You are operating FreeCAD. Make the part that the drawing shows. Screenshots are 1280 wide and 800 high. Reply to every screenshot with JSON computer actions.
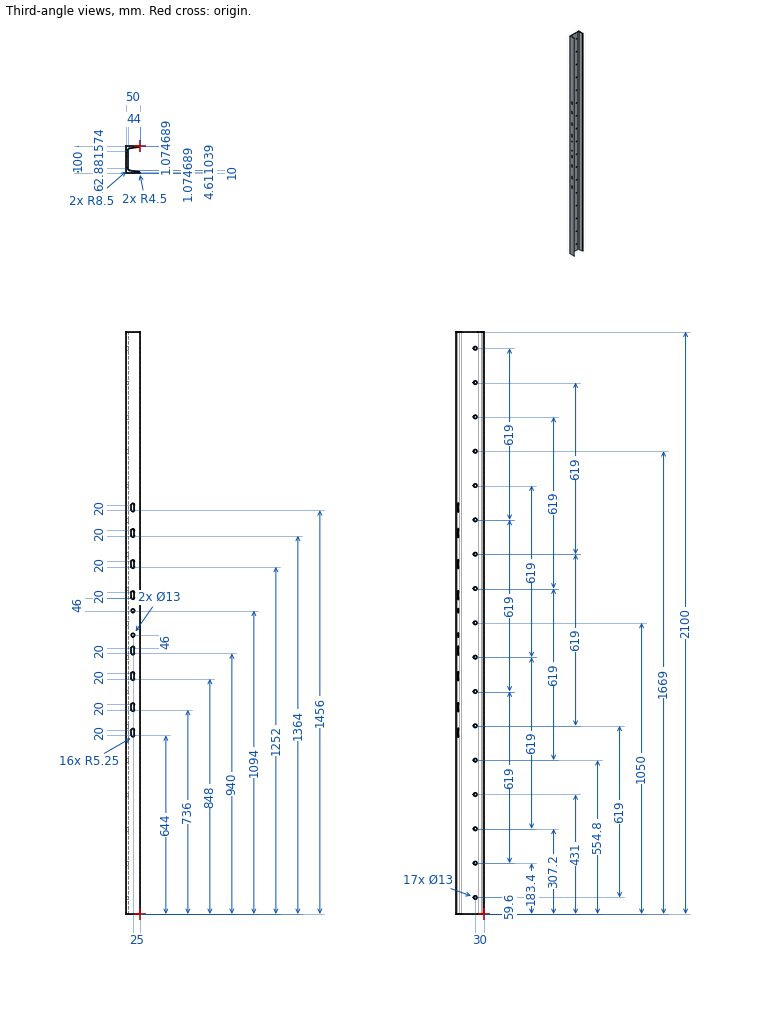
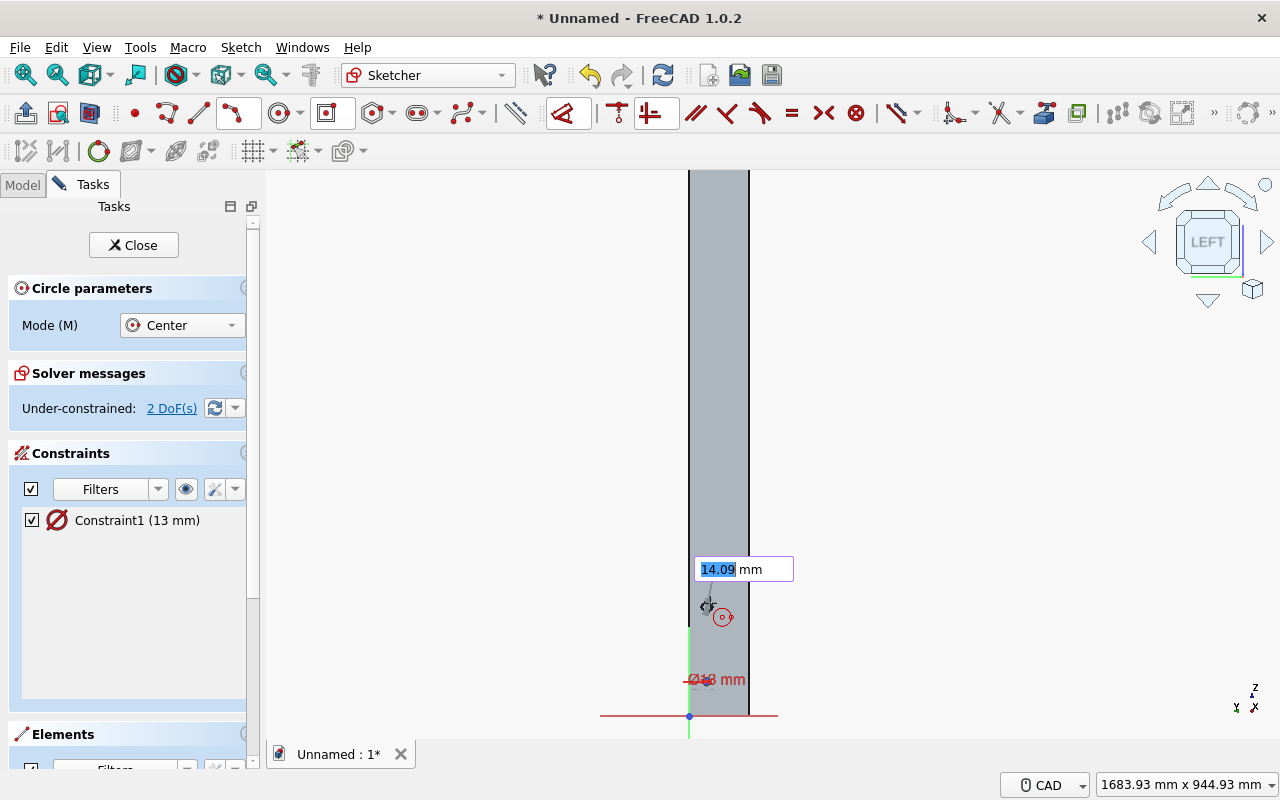
{"action": "type", "text": "13"}
{"action": "key", "text": "Return"}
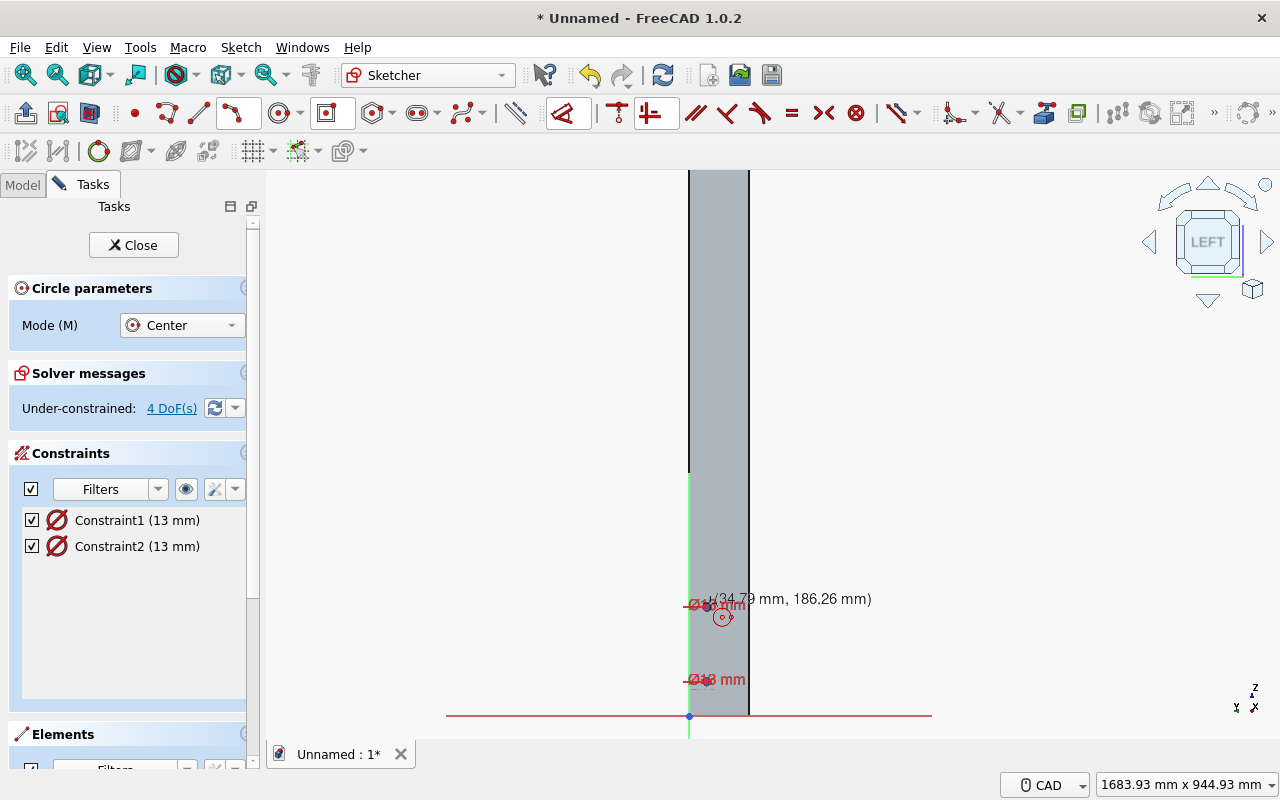
{"action": "scroll", "coordinate": [707, 531], "scroll_direction": "up", "scroll_amount": 9}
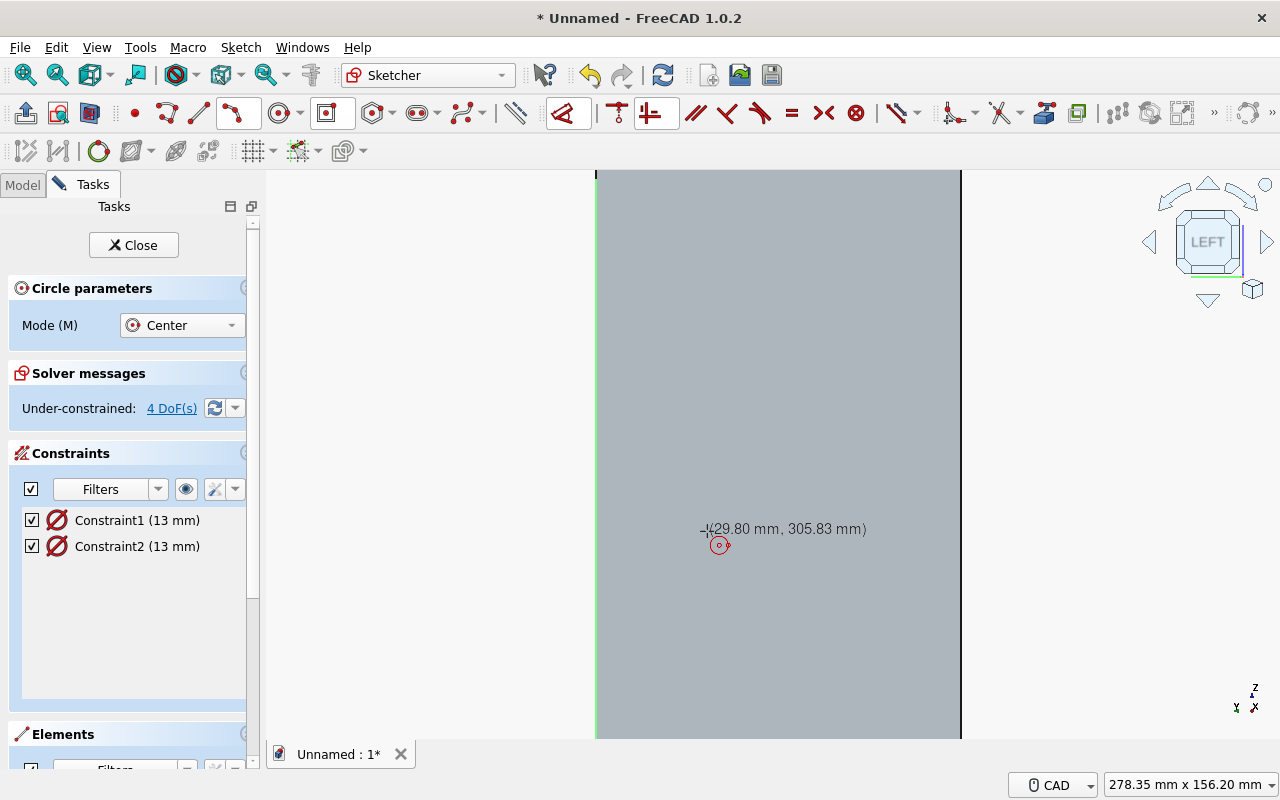
{"action": "scroll", "coordinate": [707, 587], "scroll_direction": "down", "scroll_amount": 15}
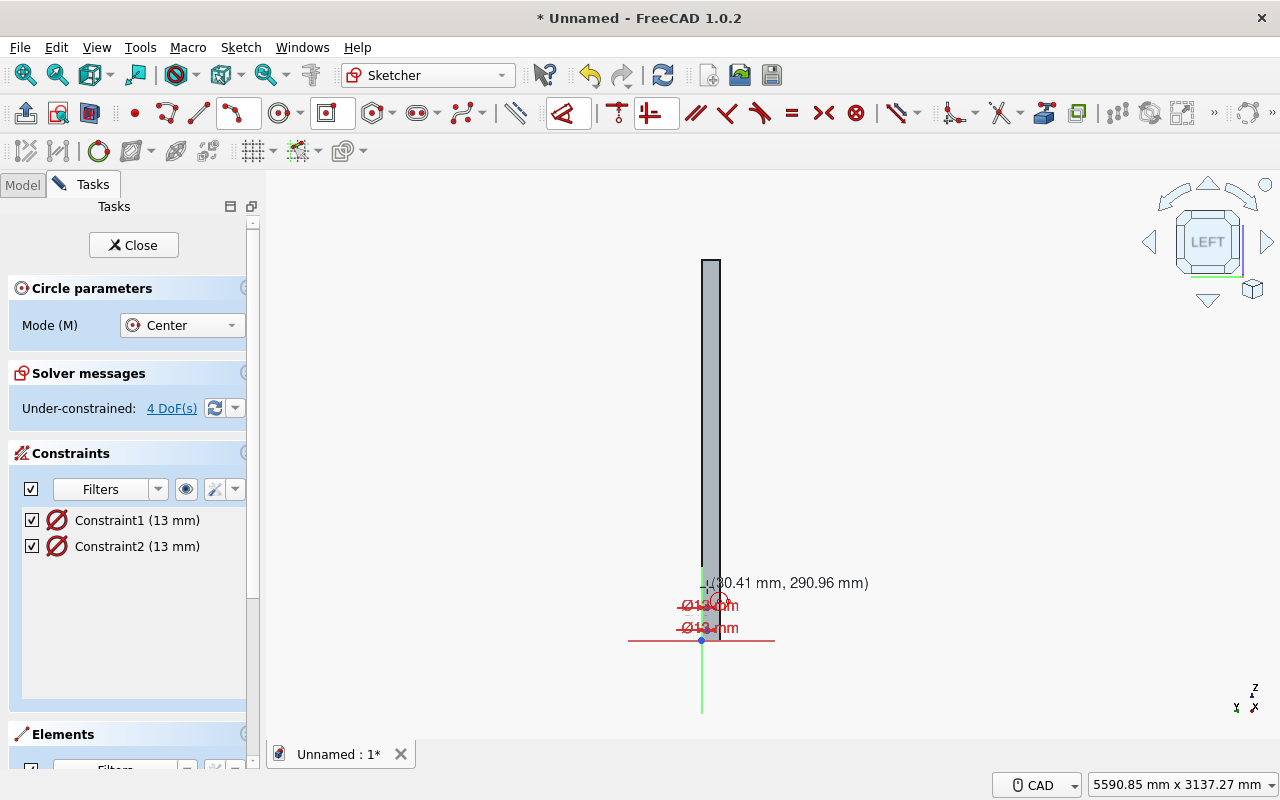
{"action": "scroll", "coordinate": [707, 585], "scroll_direction": "up", "scroll_amount": 6}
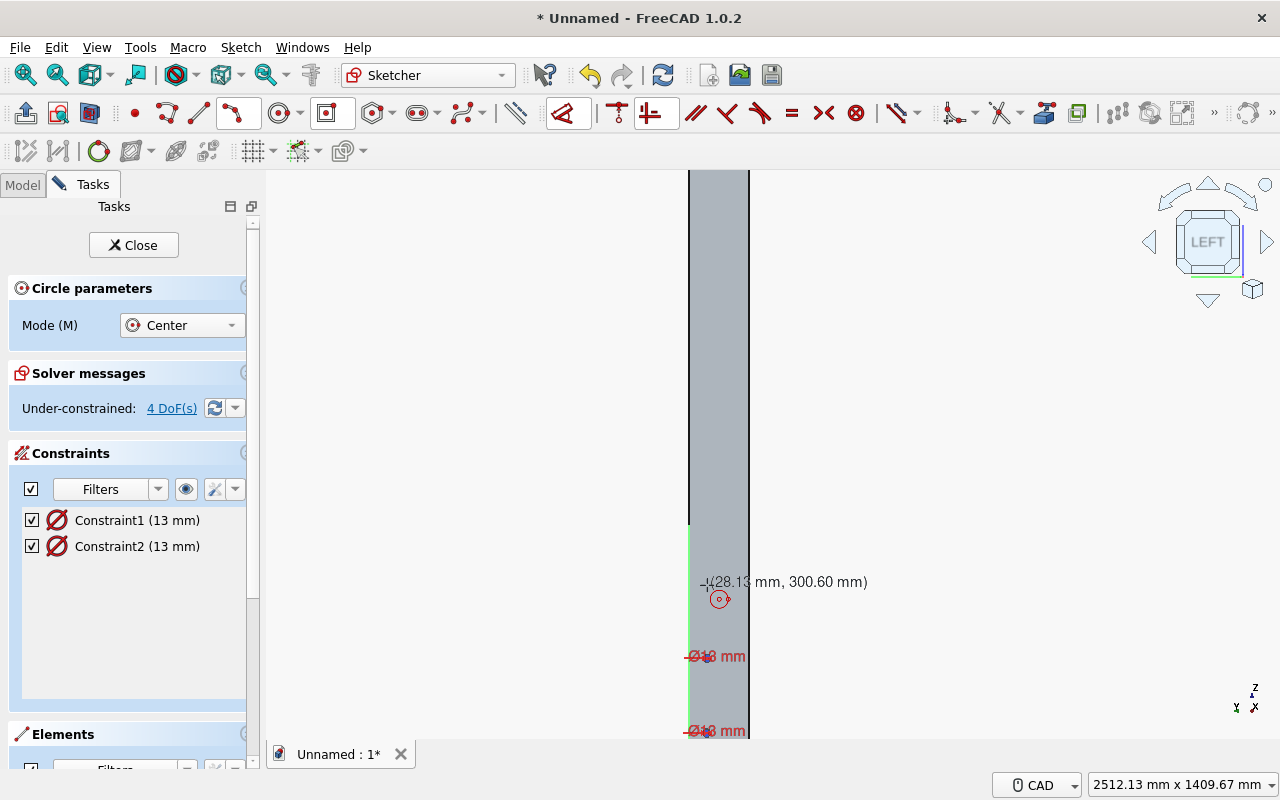
{"action": "left_click", "coordinate": [707, 583]}
{"action": "mouse_move", "coordinate": [710, 580]}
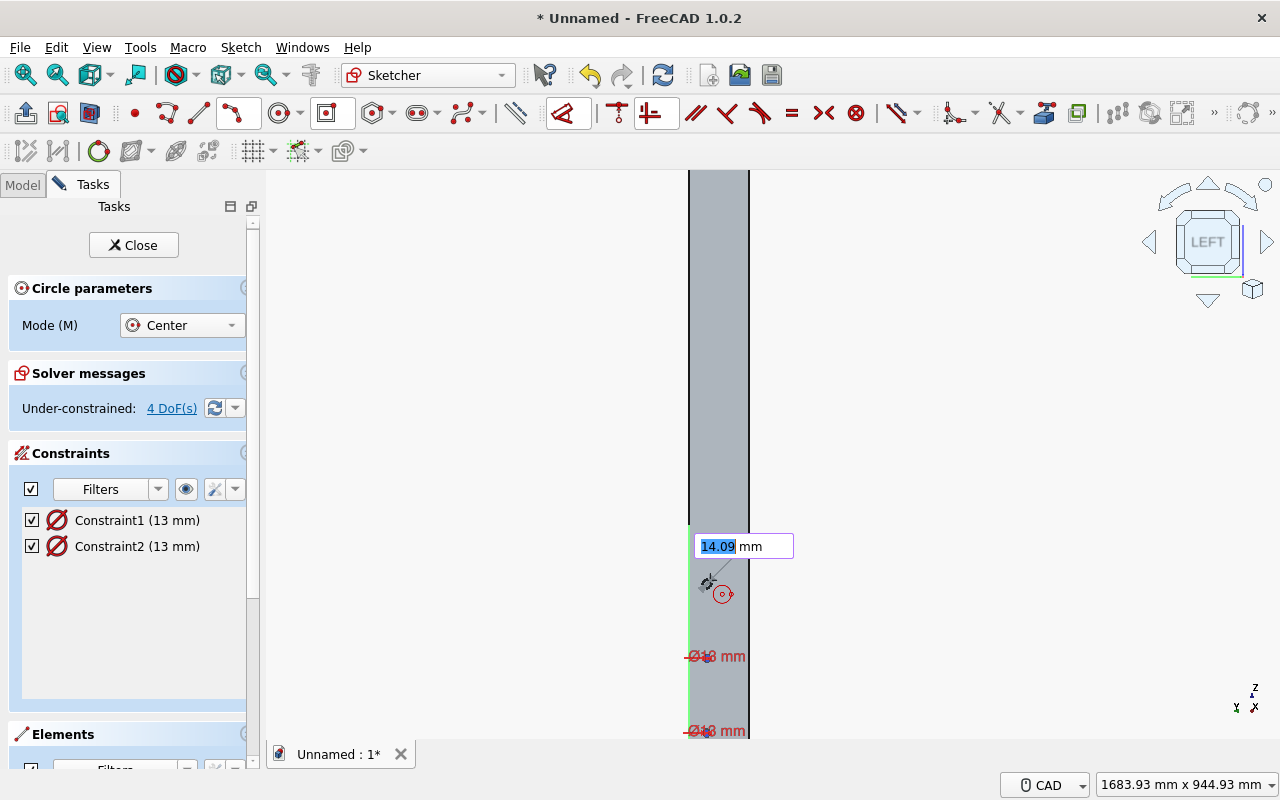
{"action": "type", "text": "13"}
{"action": "key", "text": "Return"}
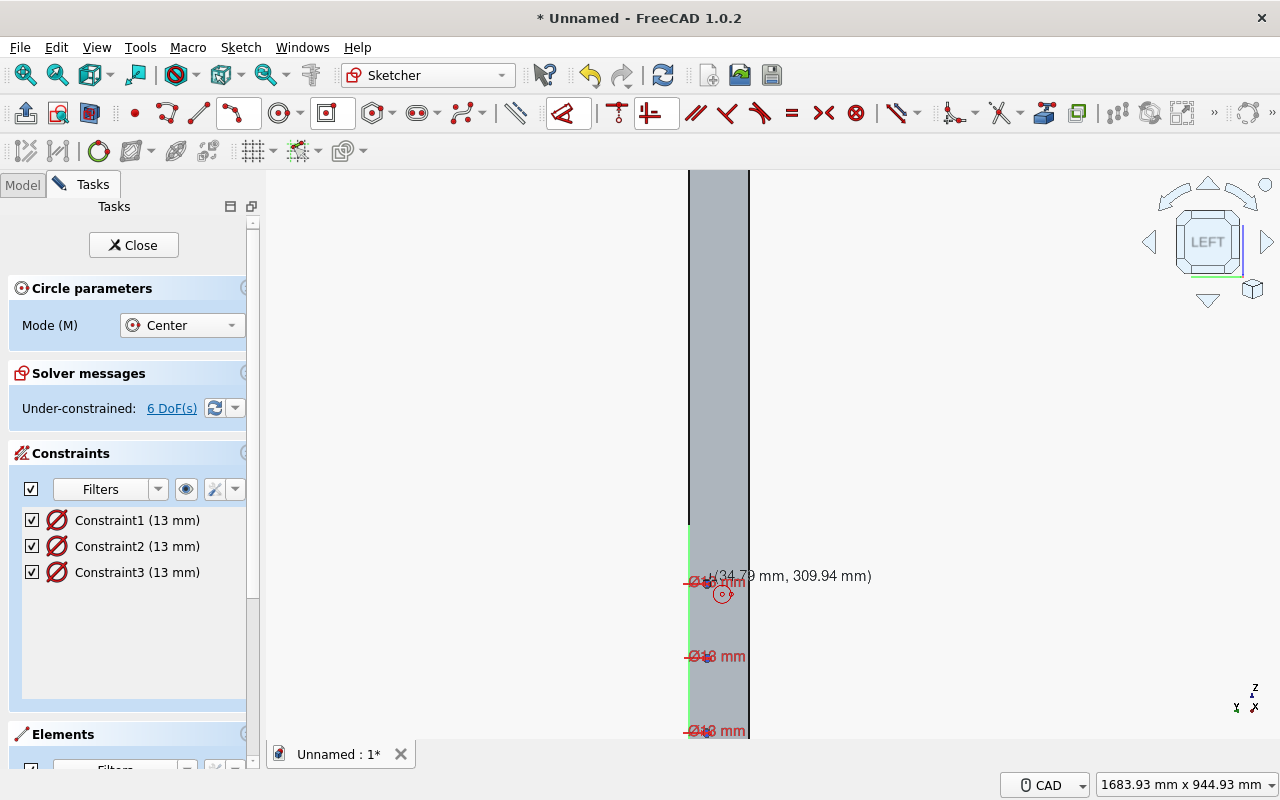
{"action": "scroll", "coordinate": [707, 508], "scroll_direction": "up", "scroll_amount": 9}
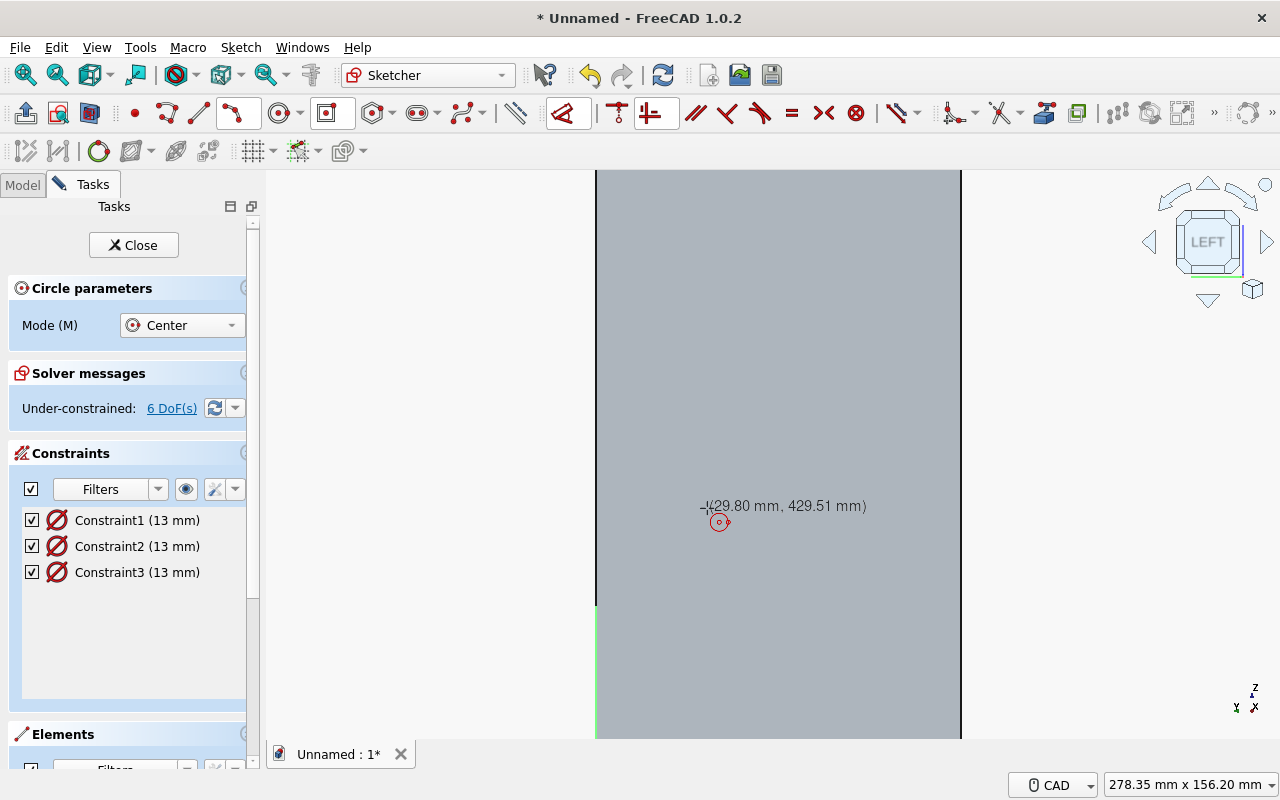
{"action": "scroll", "coordinate": [707, 565], "scroll_direction": "down", "scroll_amount": 15}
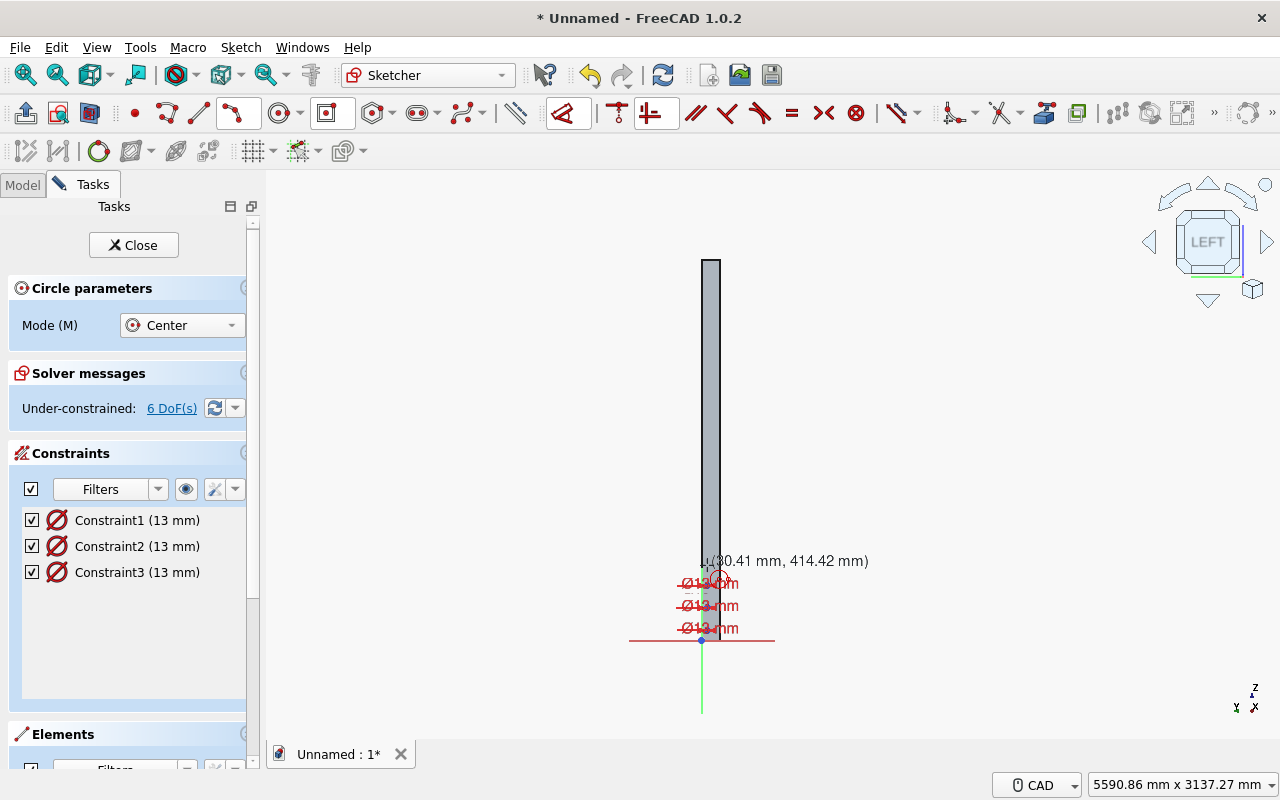
{"action": "scroll", "coordinate": [707, 563], "scroll_direction": "up", "scroll_amount": 6}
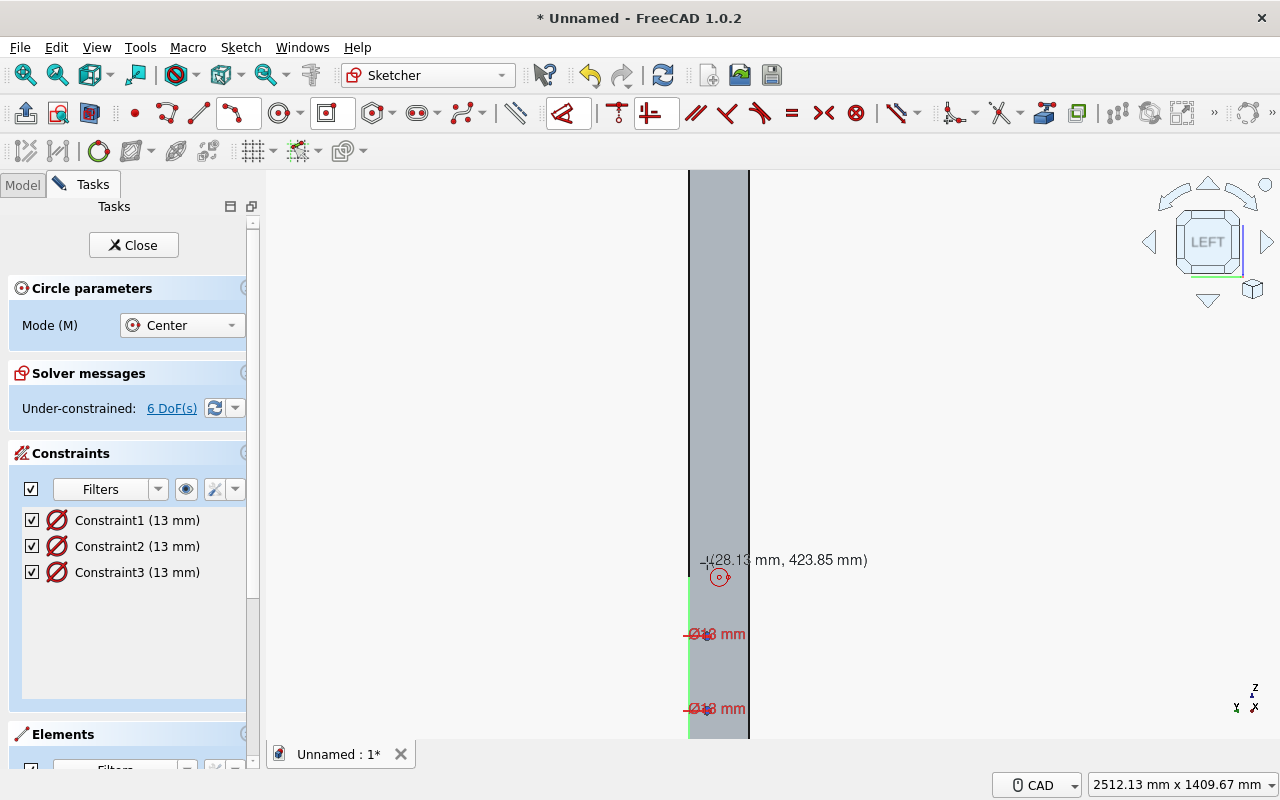
{"action": "left_click", "coordinate": [707, 560]}
{"action": "mouse_move", "coordinate": [710, 558]}